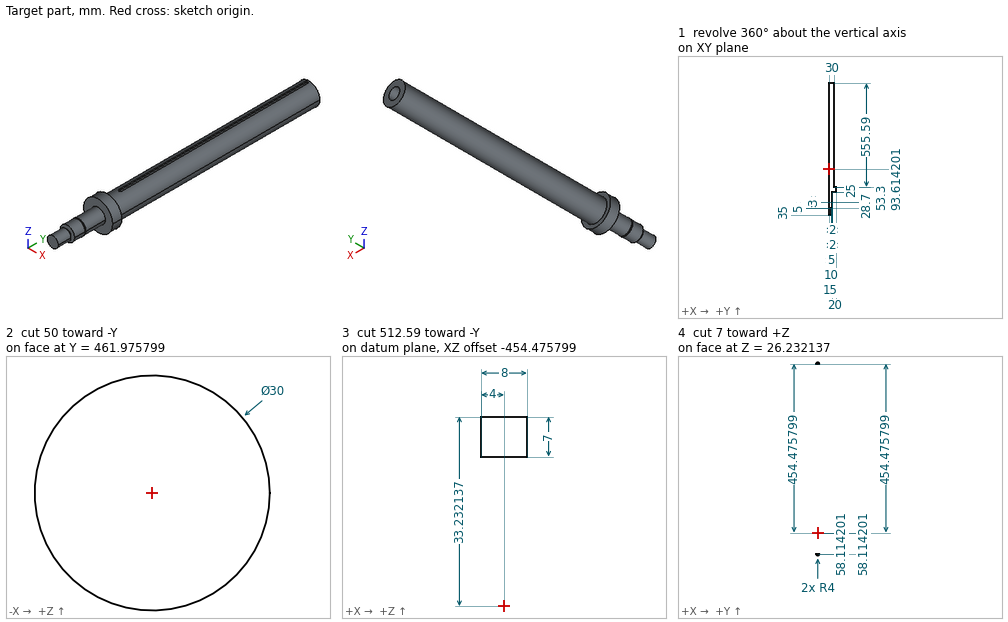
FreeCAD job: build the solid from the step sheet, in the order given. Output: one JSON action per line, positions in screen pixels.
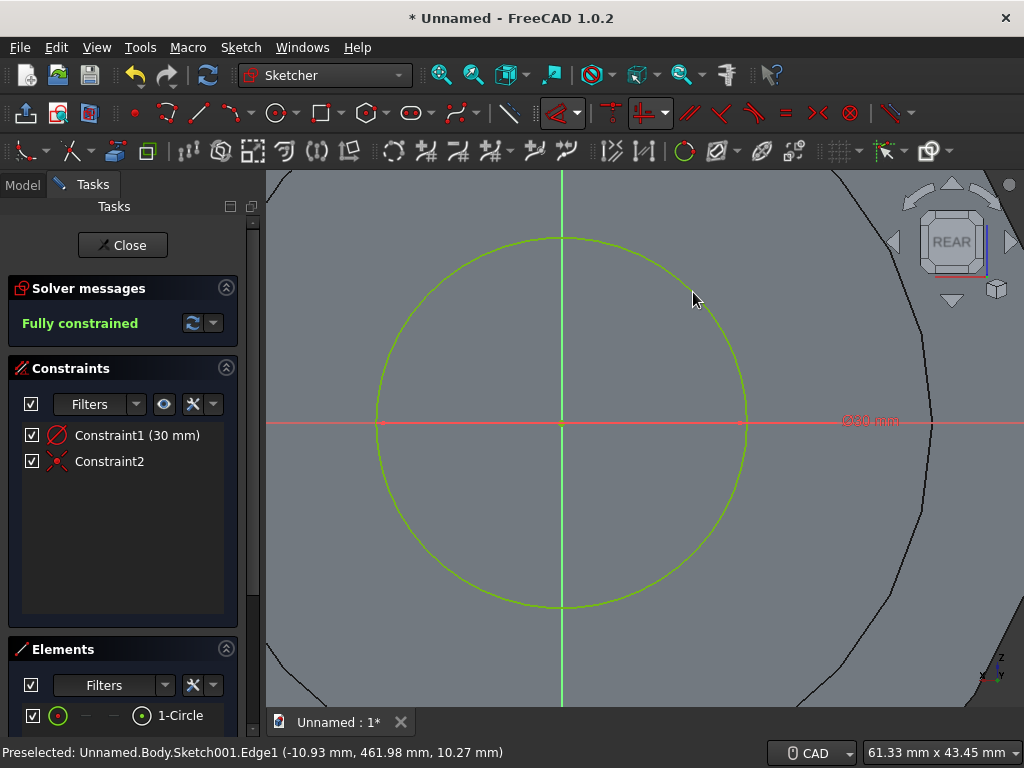
{"action": "left_click", "coordinate": [123, 245]}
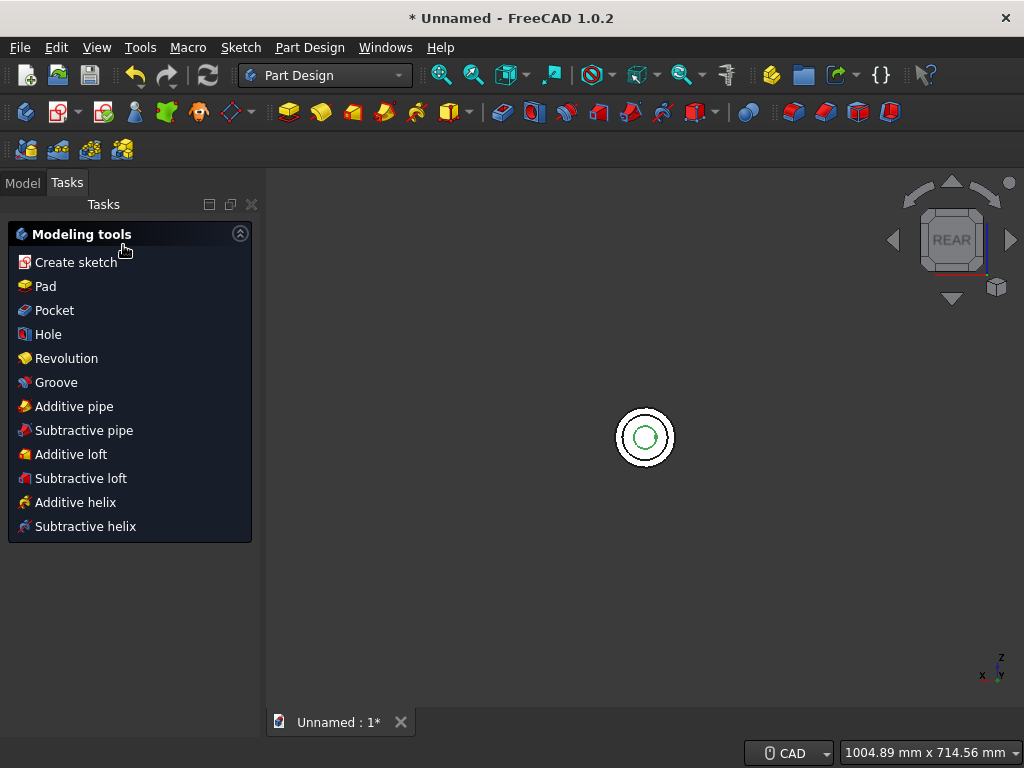
{"action": "left_click", "coordinate": [504, 112]}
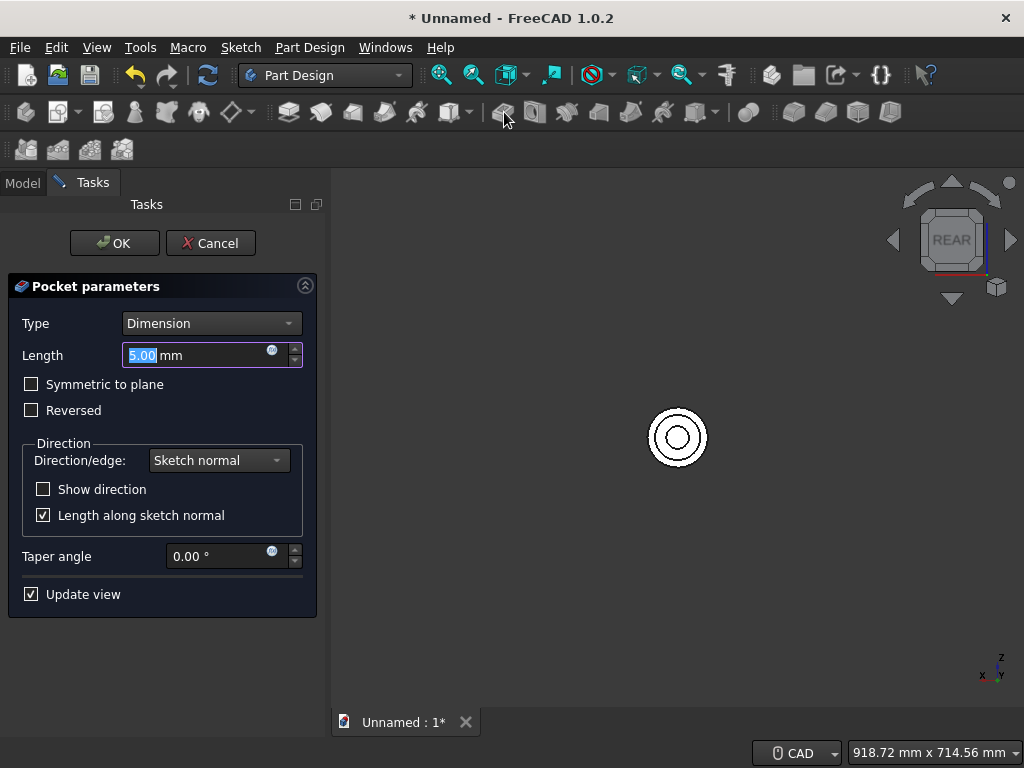
{"action": "type", "text": "50"}
{"action": "key", "text": "Tab"}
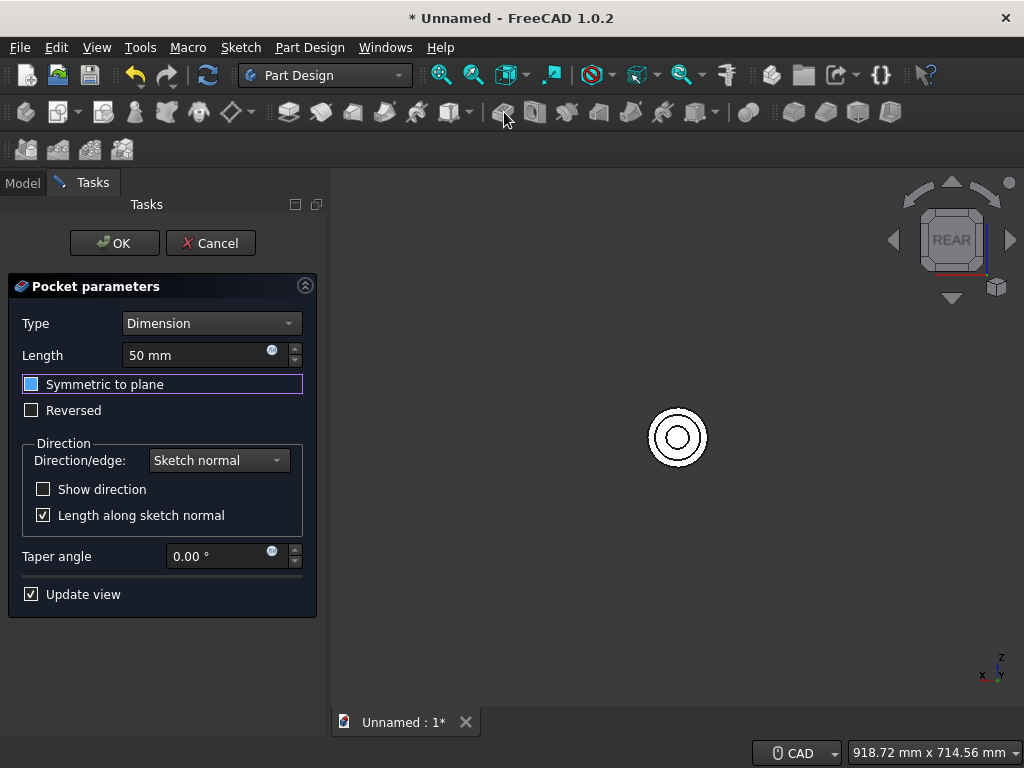
{"action": "left_click", "coordinate": [115, 243]}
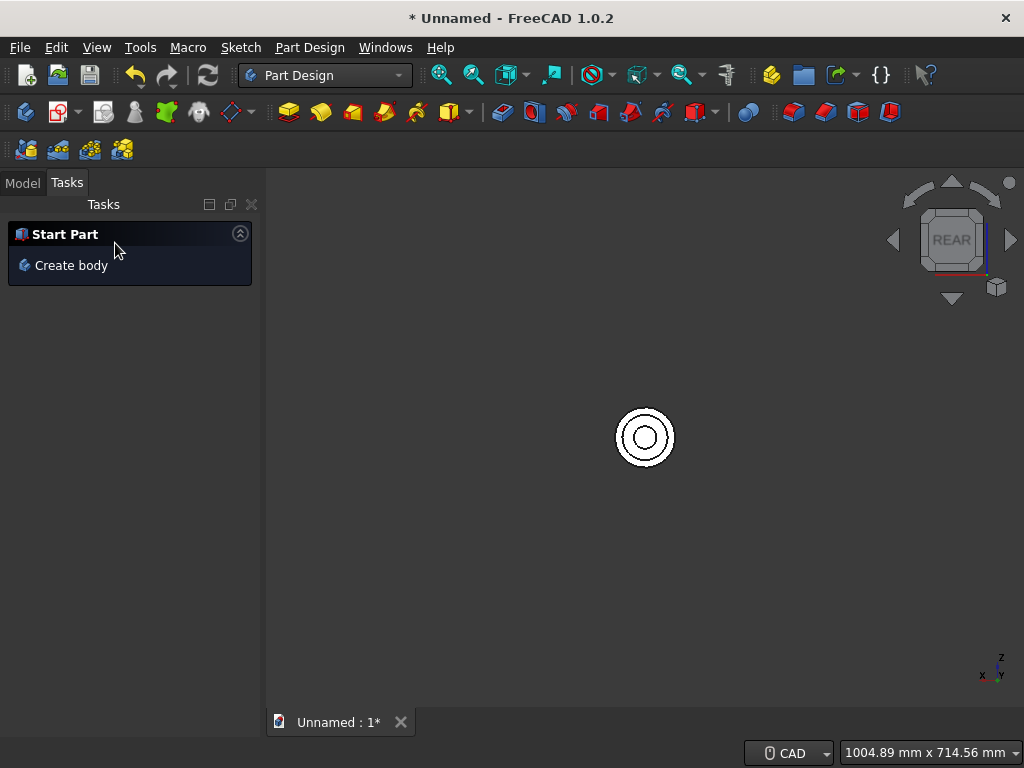
{"action": "key", "text": "v f"}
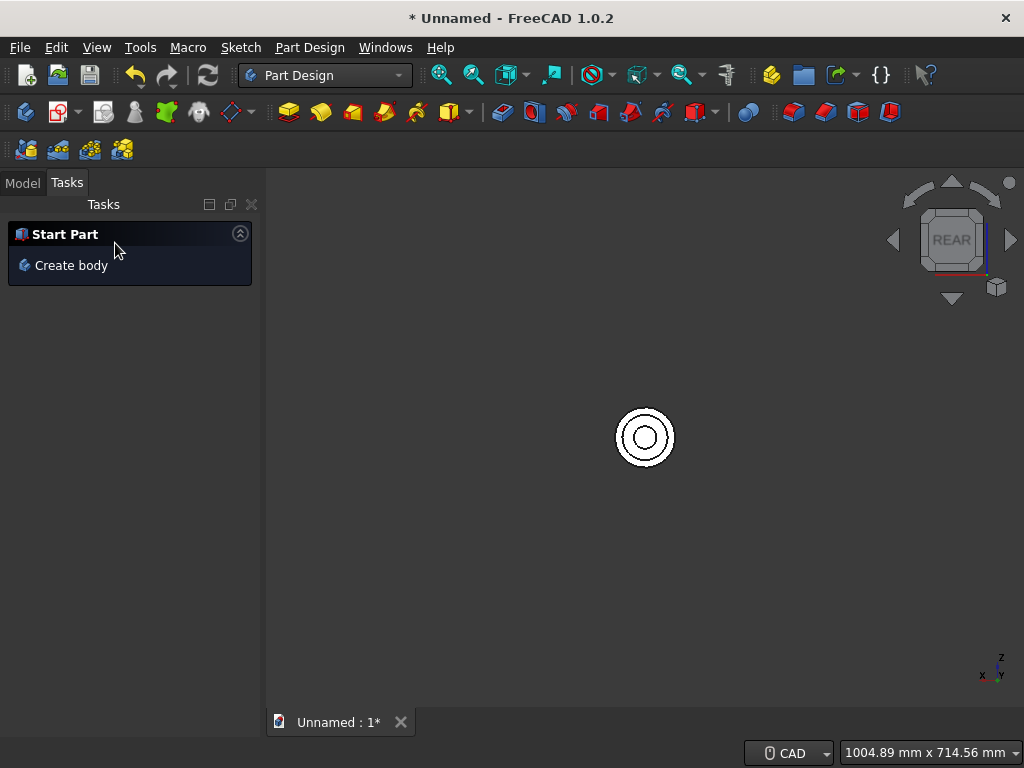
{"action": "left_click", "coordinate": [23, 182]}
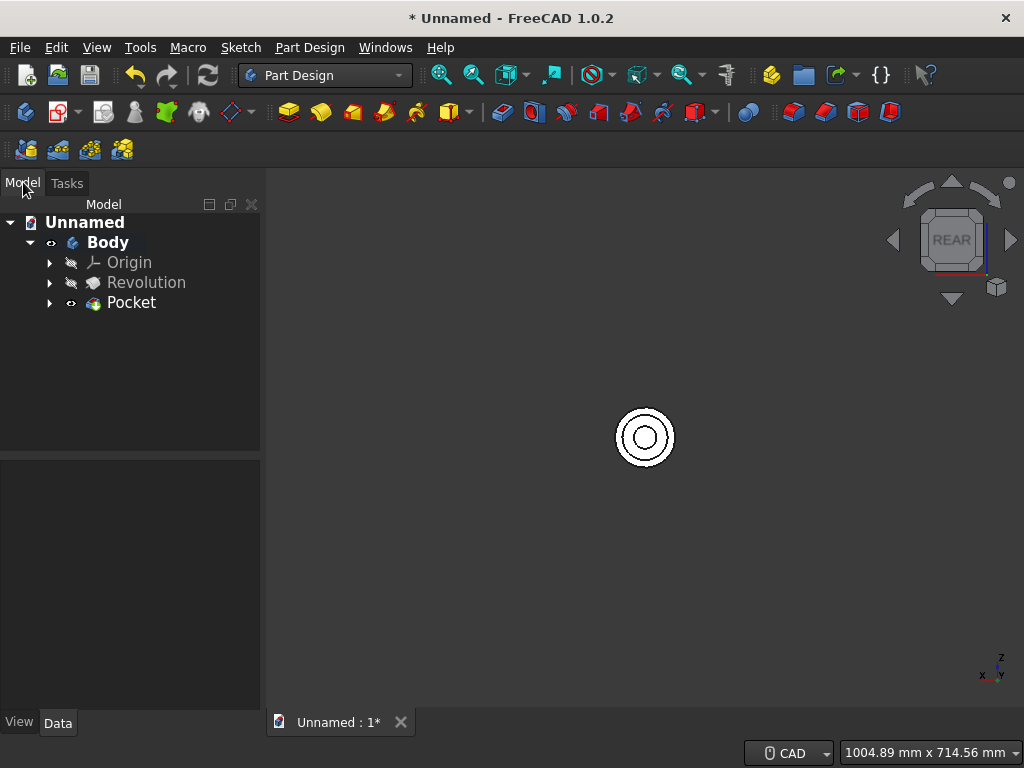
{"action": "left_click", "coordinate": [50, 263]}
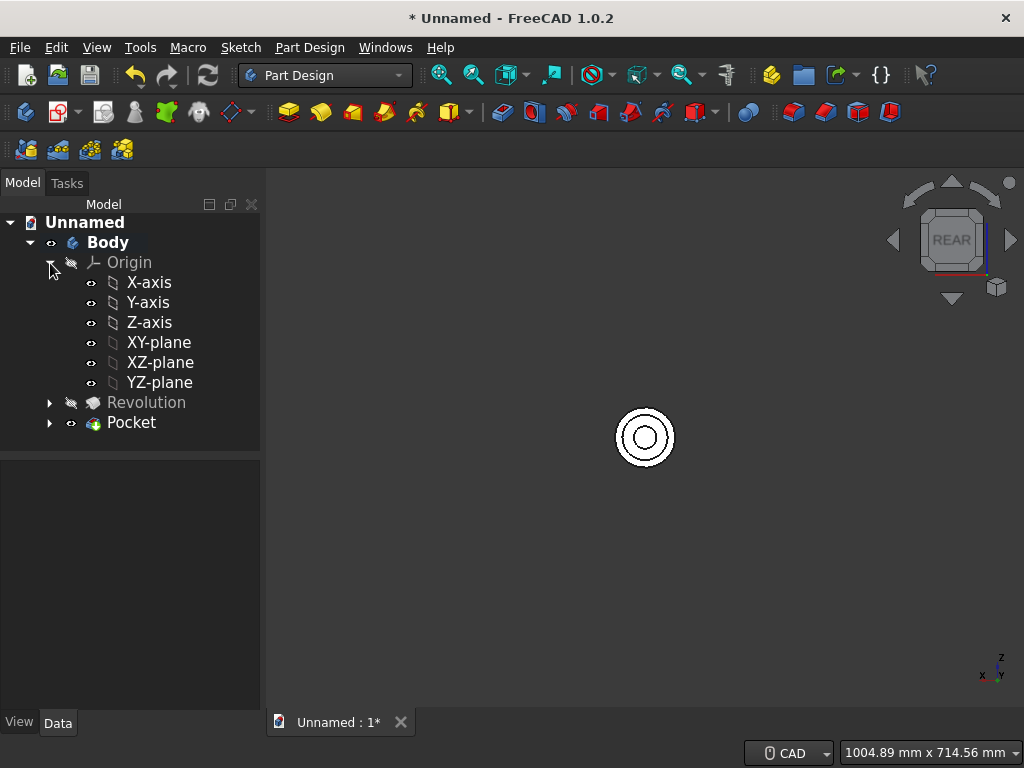
{"action": "left_click", "coordinate": [136, 363]}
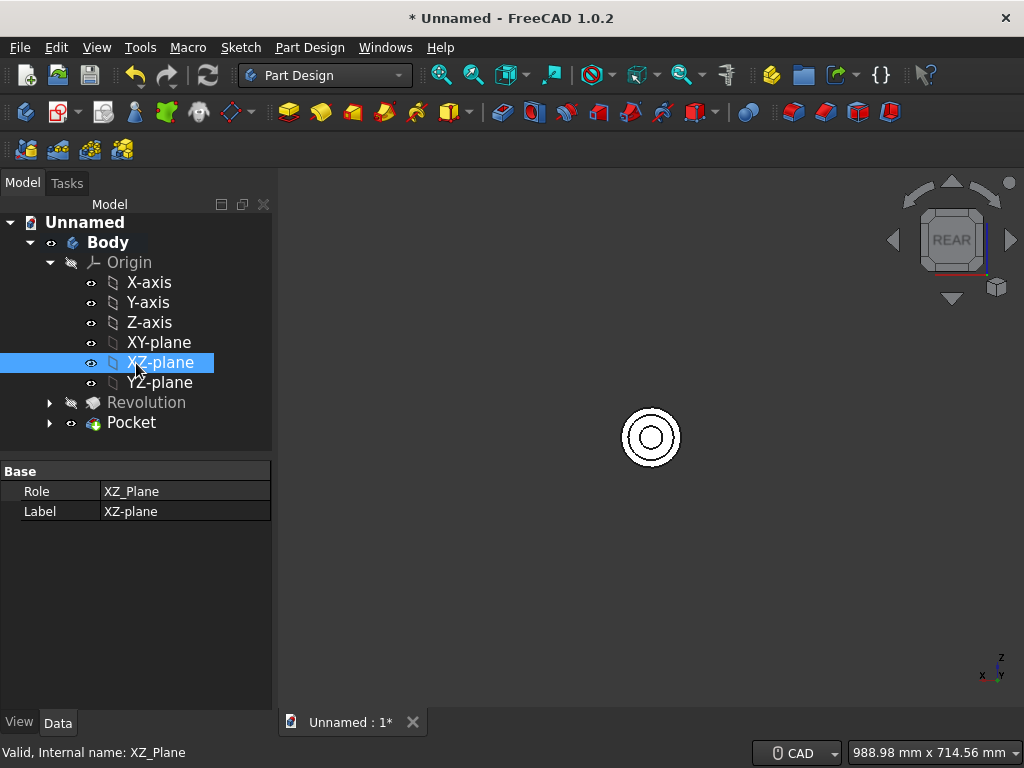
{"action": "left_click", "coordinate": [232, 112]}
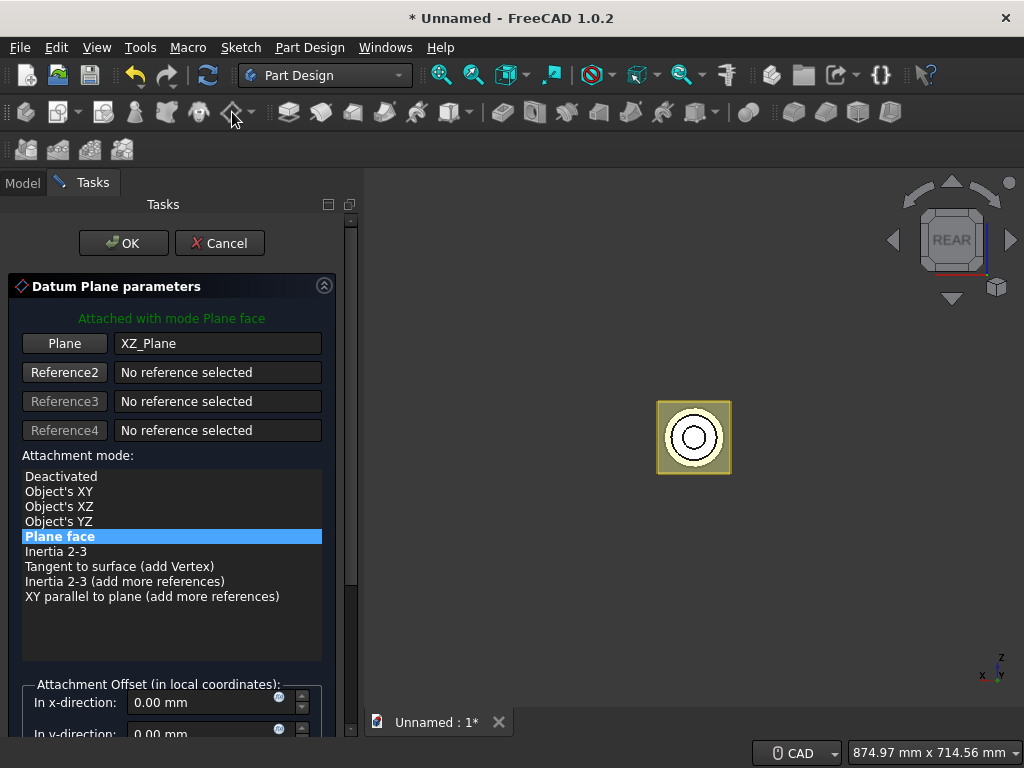
{"action": "scroll", "coordinate": [351, 475], "scroll_direction": "down", "scroll_amount": 2}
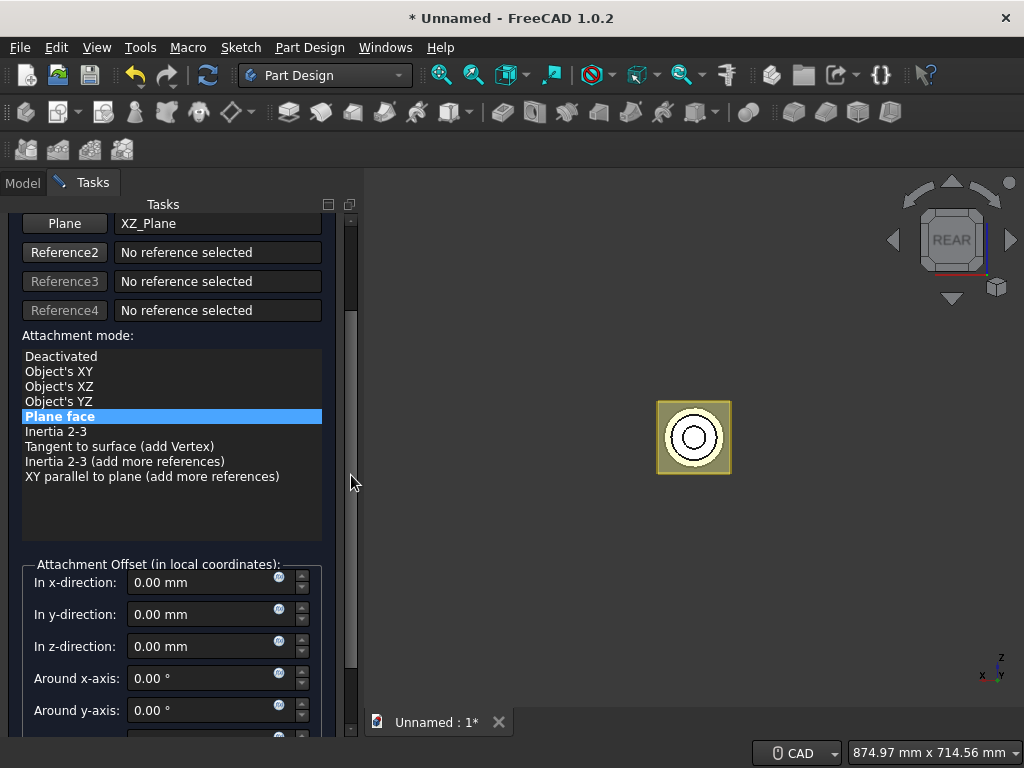
{"action": "triple_click", "coordinate": [210, 646]}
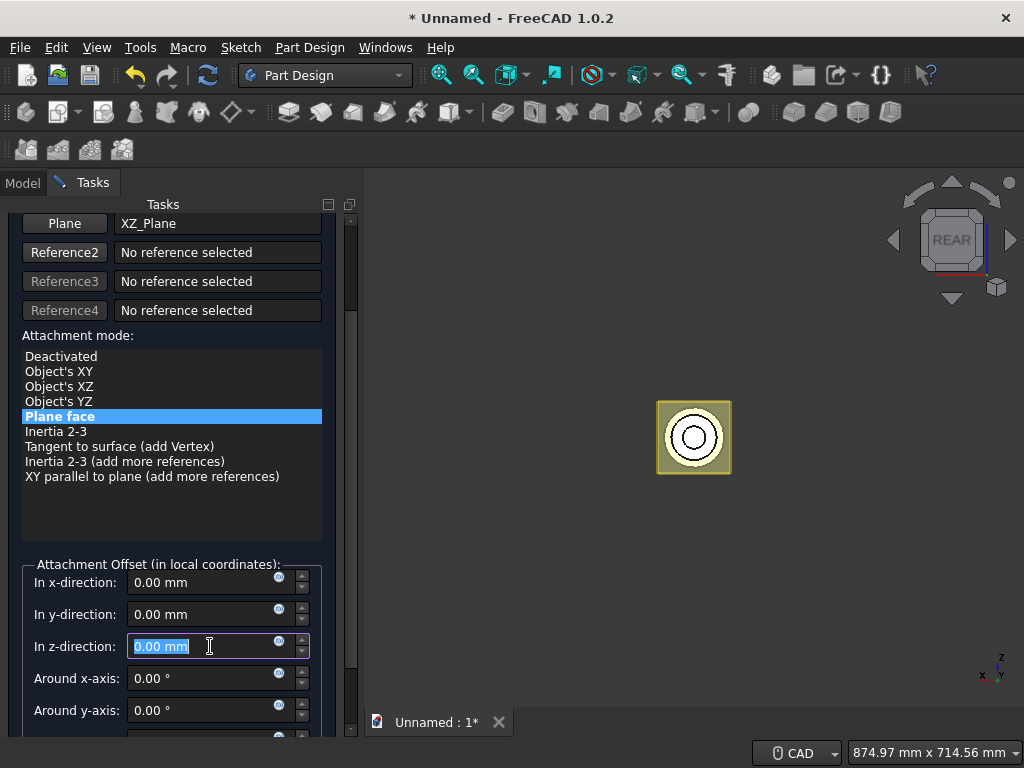
{"action": "type", "text": "-454.475799"}
{"action": "key", "text": "Tab"}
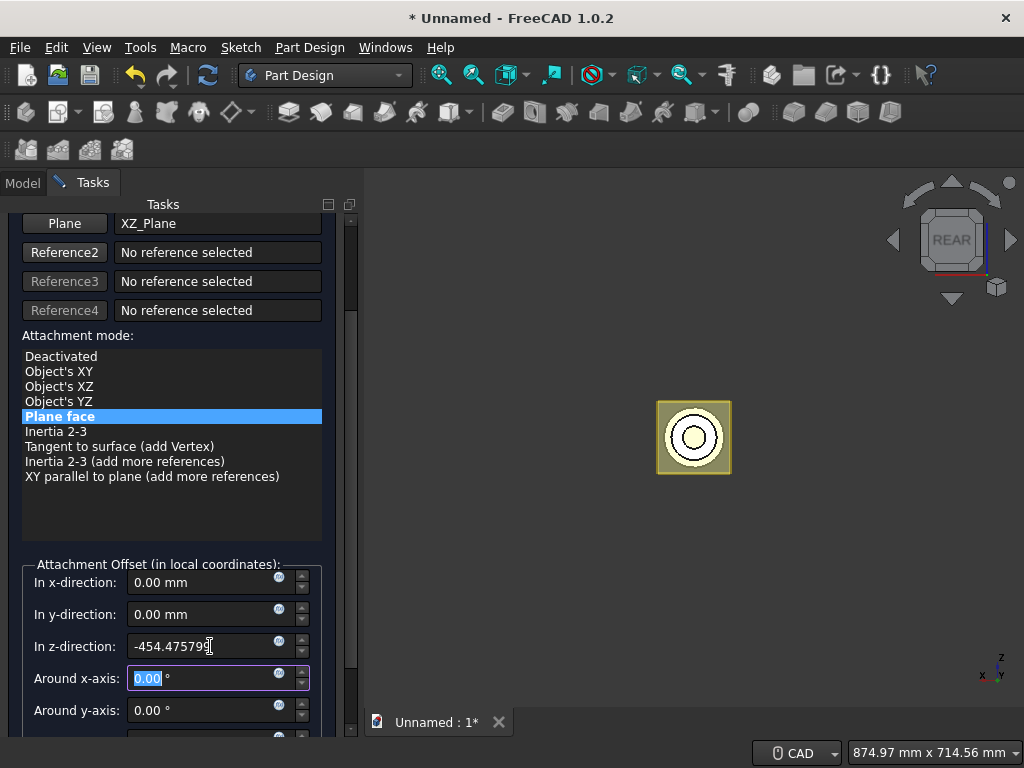
{"action": "scroll", "coordinate": [351, 475], "scroll_direction": "up", "scroll_amount": 3}